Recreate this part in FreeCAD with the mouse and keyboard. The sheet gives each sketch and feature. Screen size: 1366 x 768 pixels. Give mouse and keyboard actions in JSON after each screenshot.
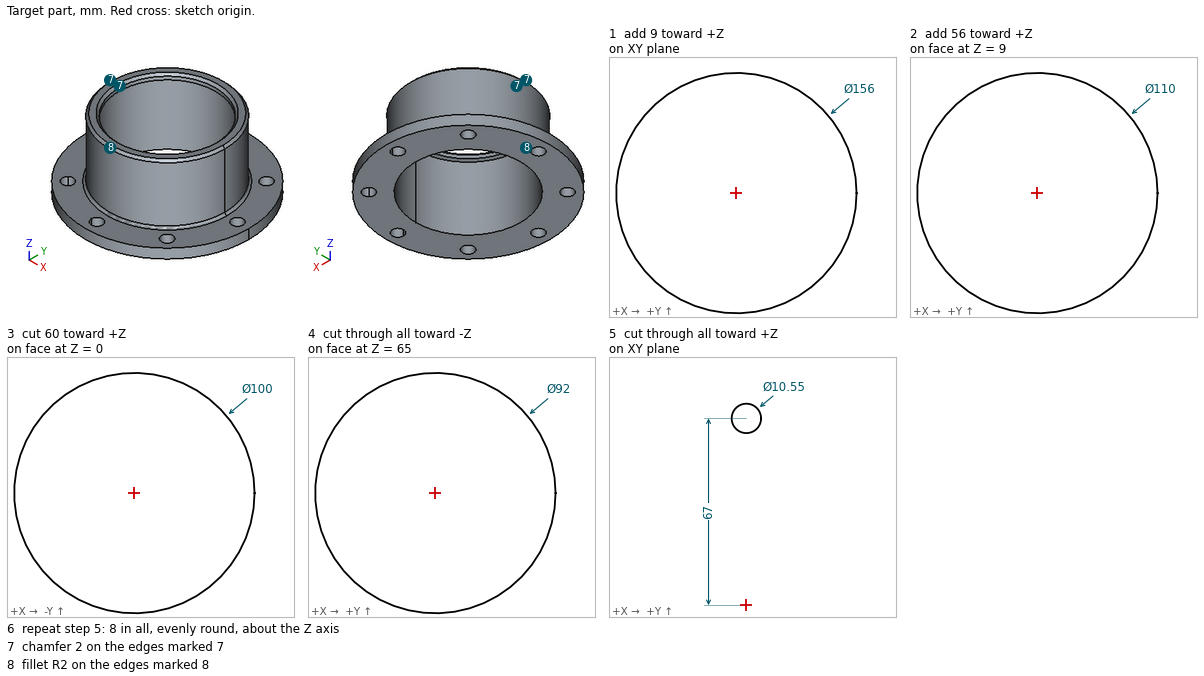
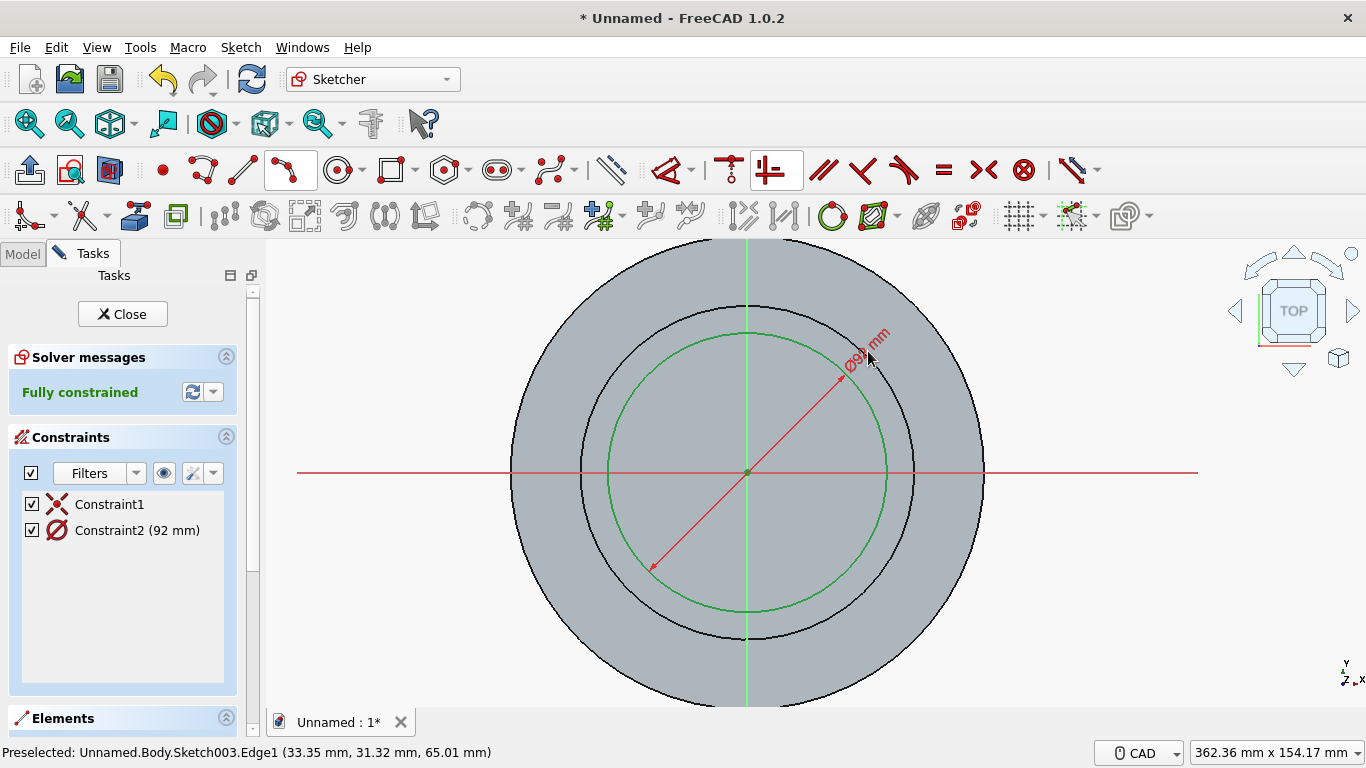
{"action": "left_click", "coordinate": [123, 314]}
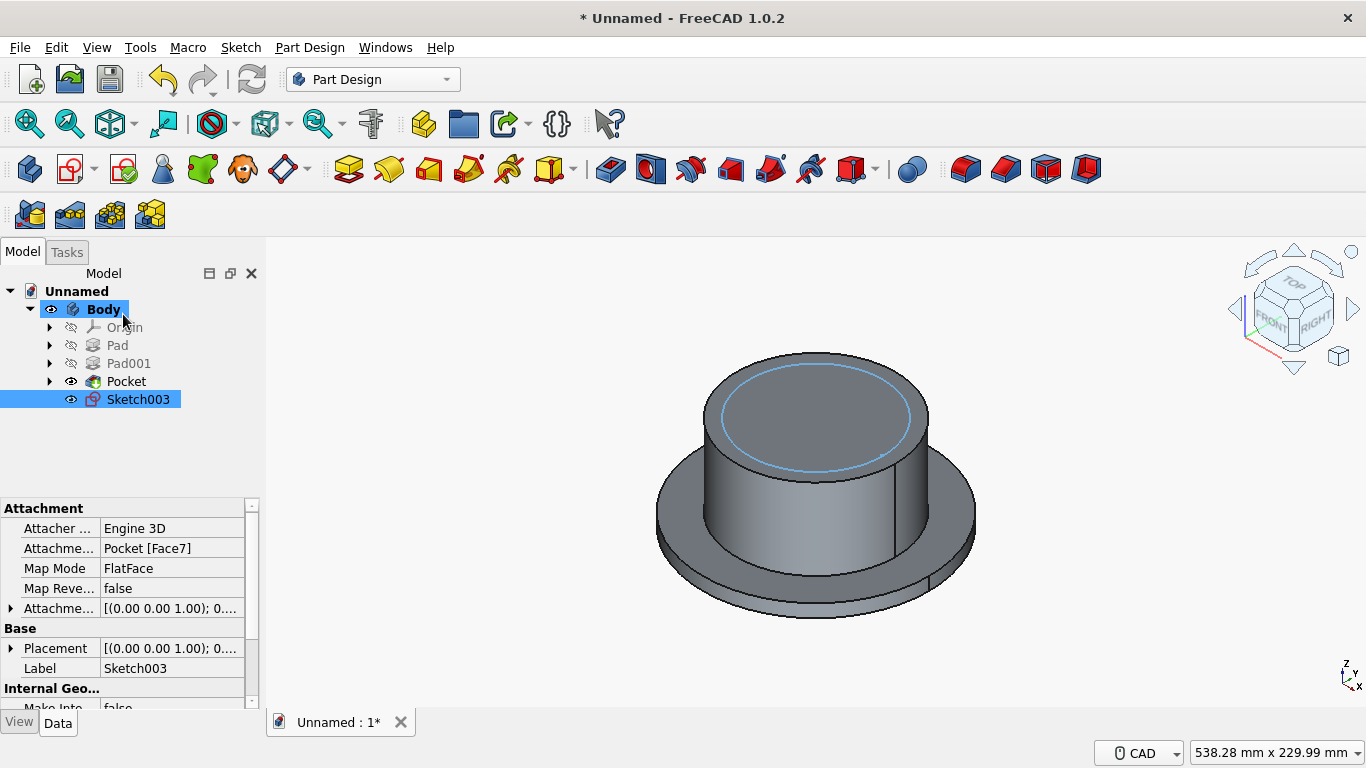
{"action": "left_click", "coordinate": [612, 170]}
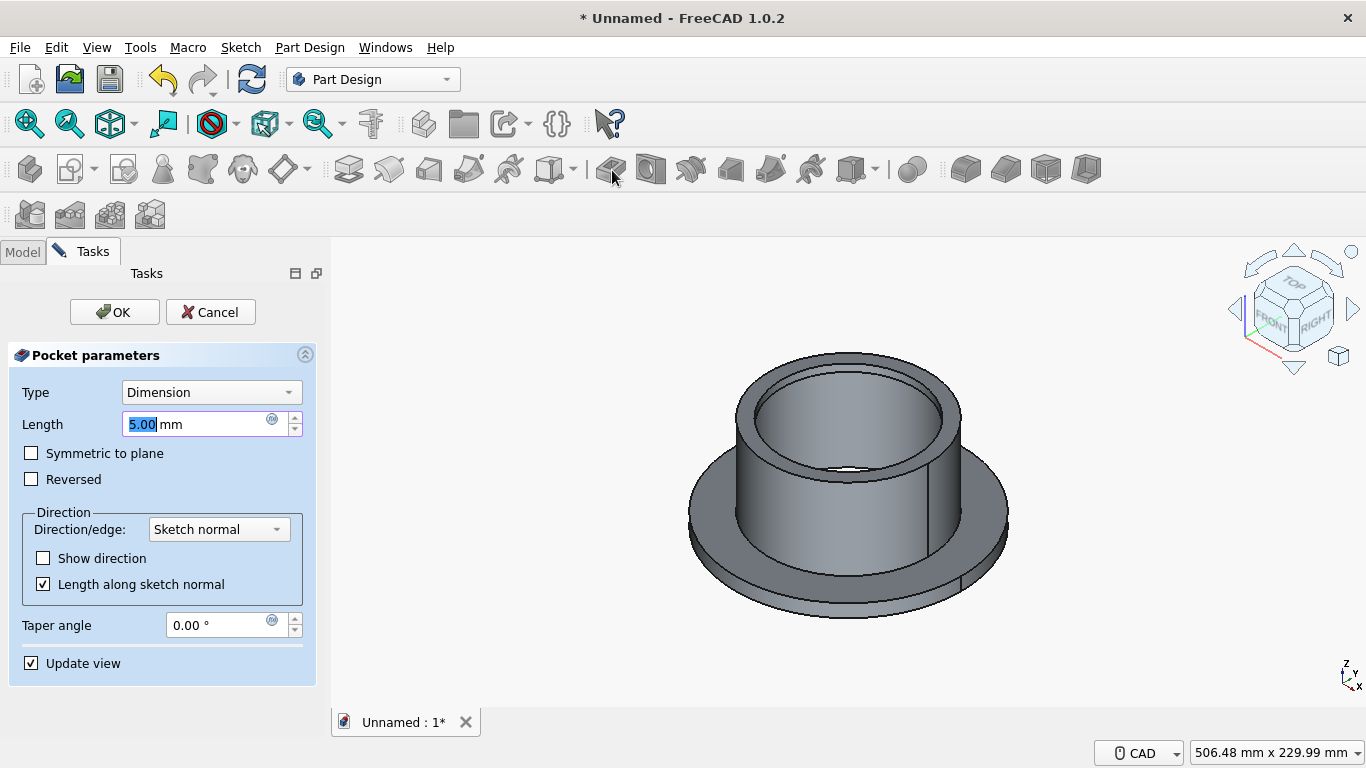
{"action": "left_click", "coordinate": [212, 392]}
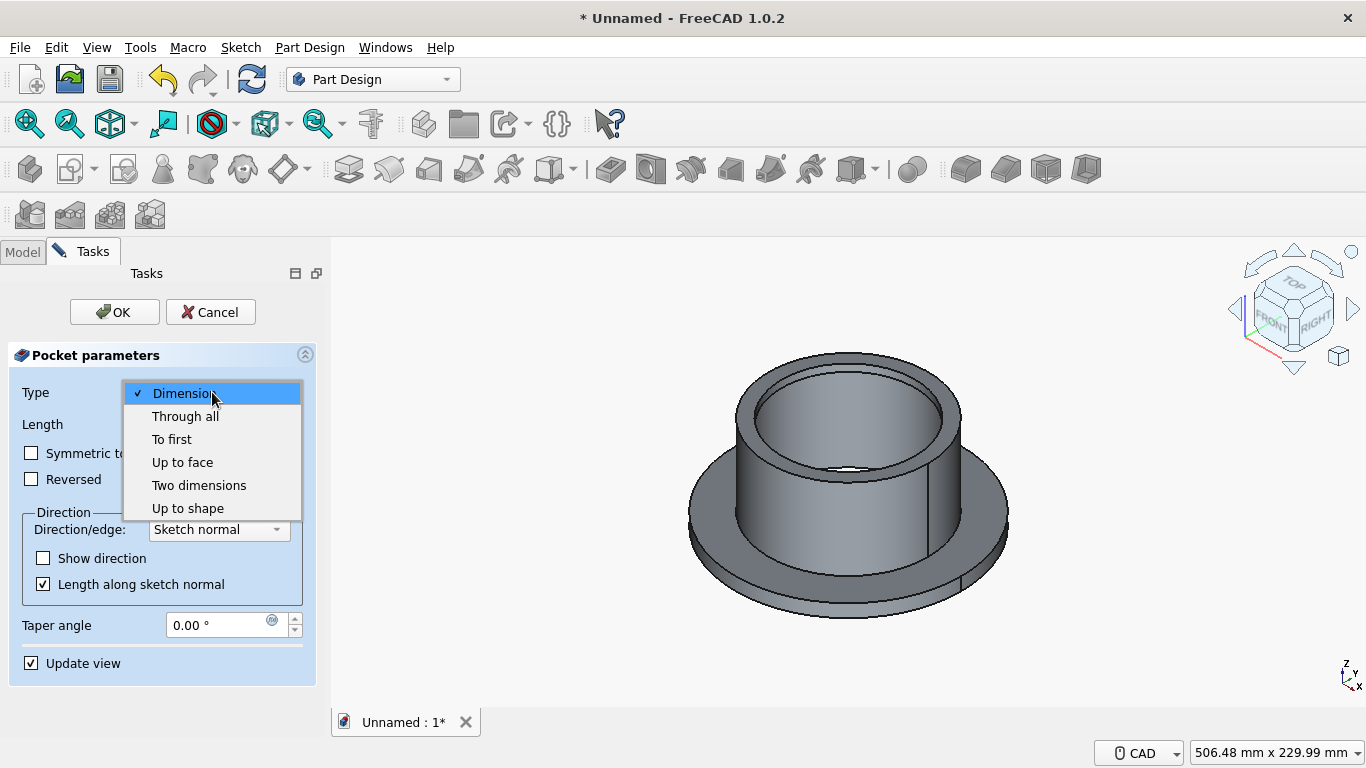
{"action": "left_click", "coordinate": [212, 416]}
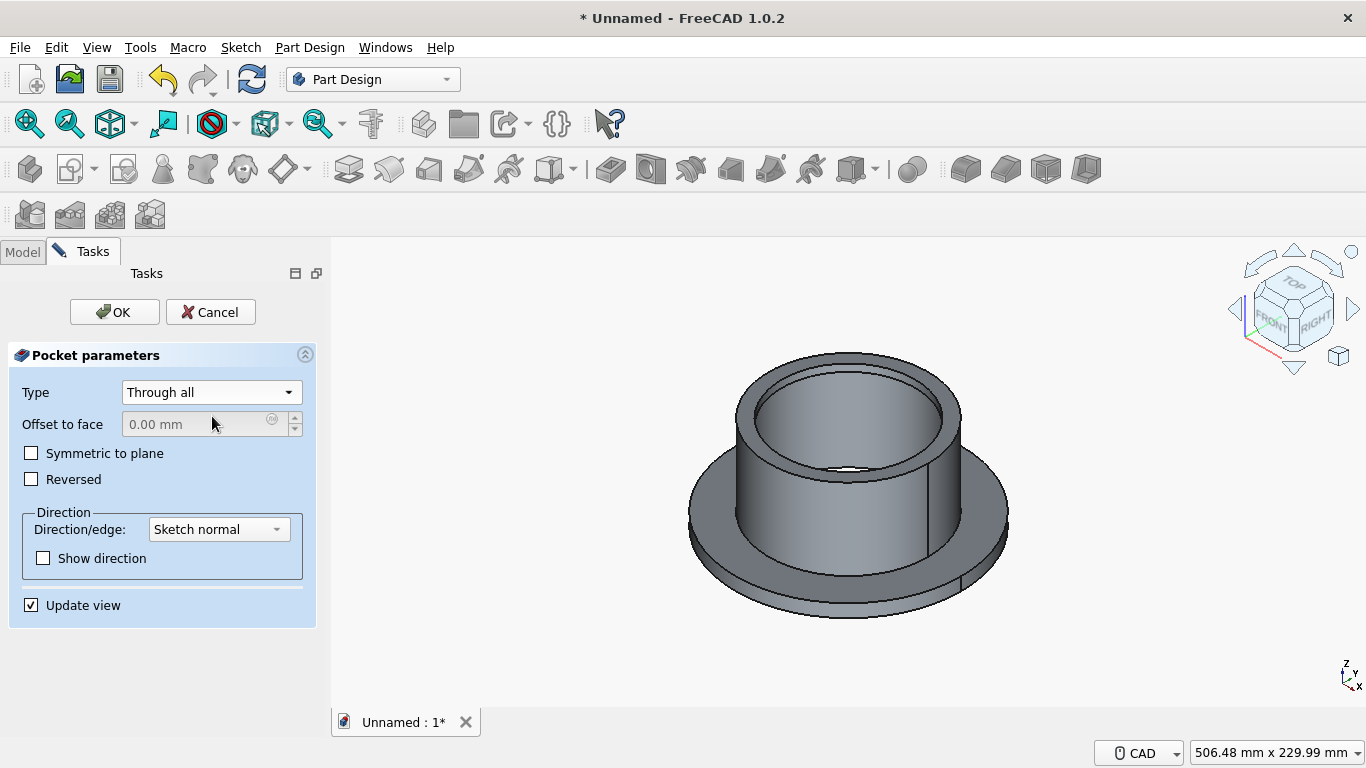
{"action": "left_click", "coordinate": [115, 312]}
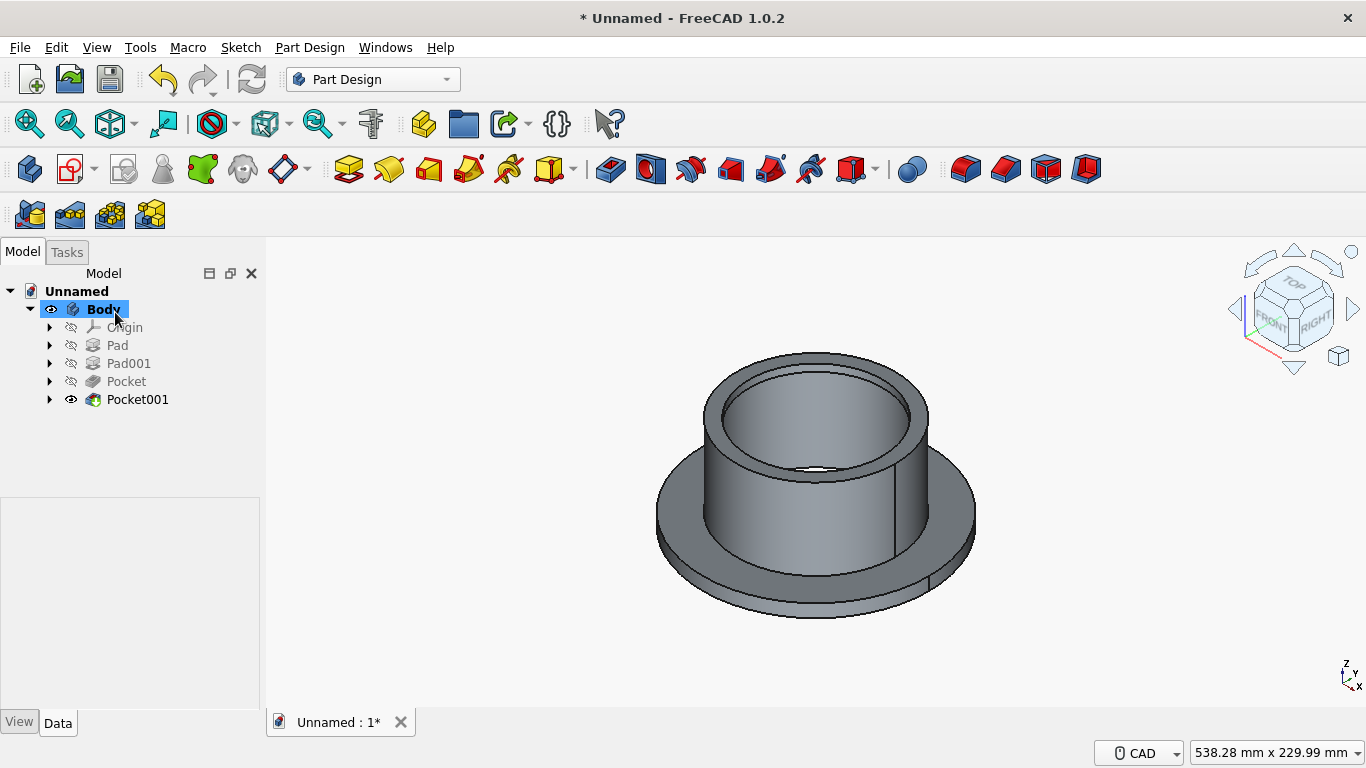
{"action": "left_click", "coordinate": [70, 170]}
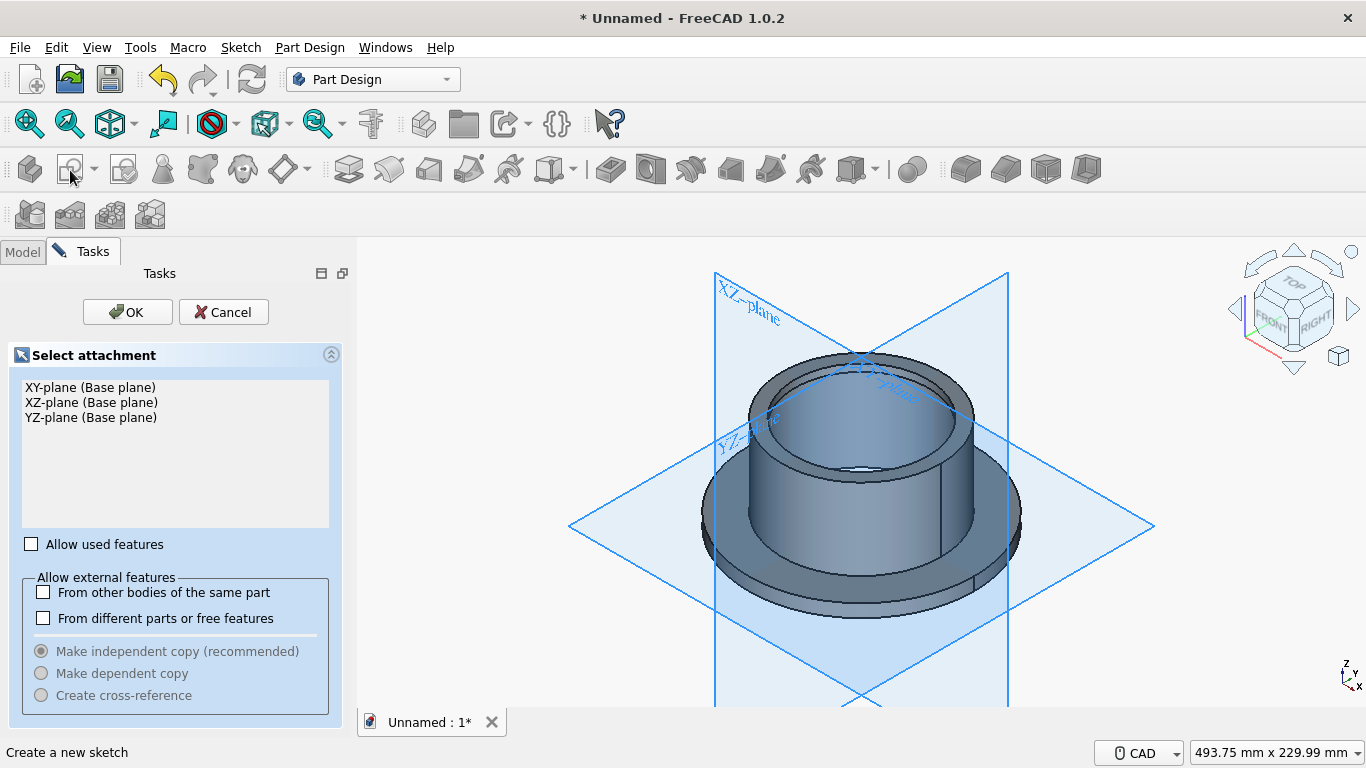
{"action": "left_click", "coordinate": [82, 388]}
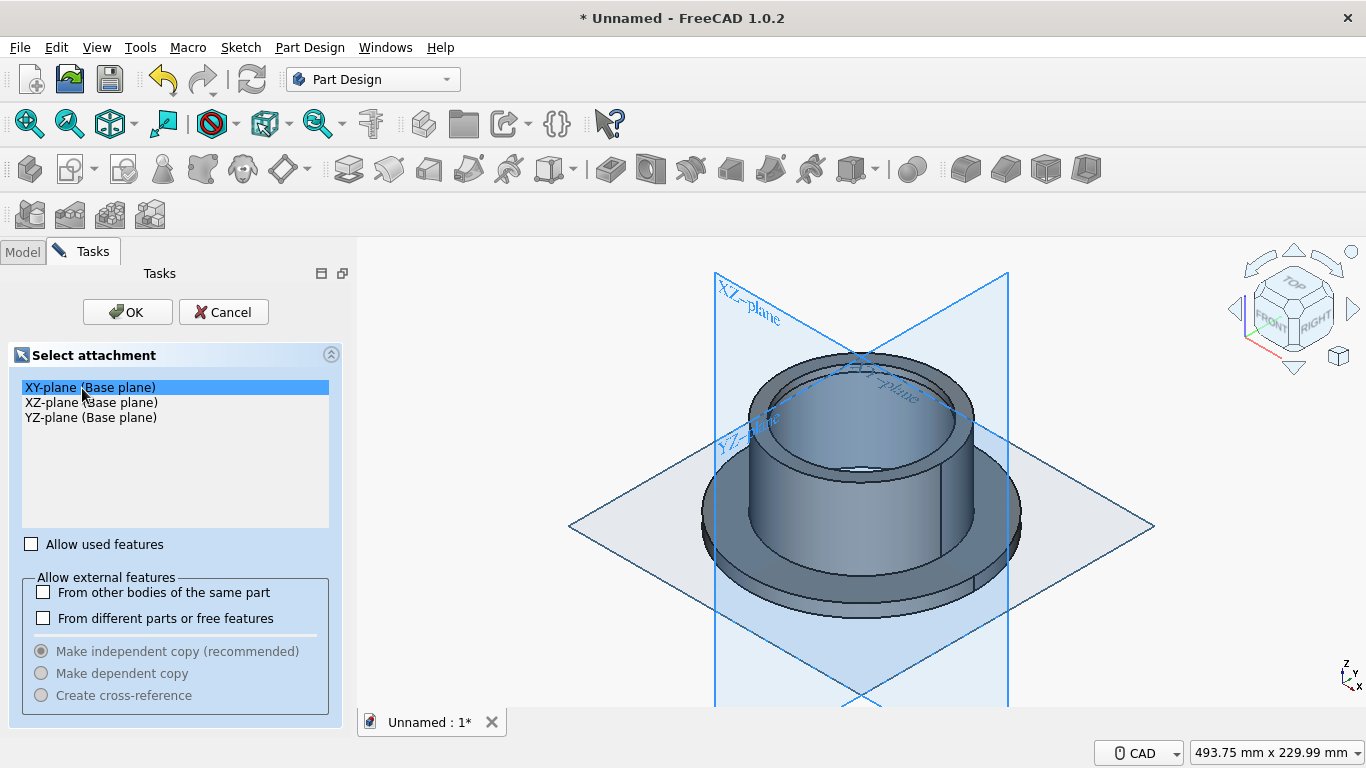
{"action": "left_click", "coordinate": [128, 312]}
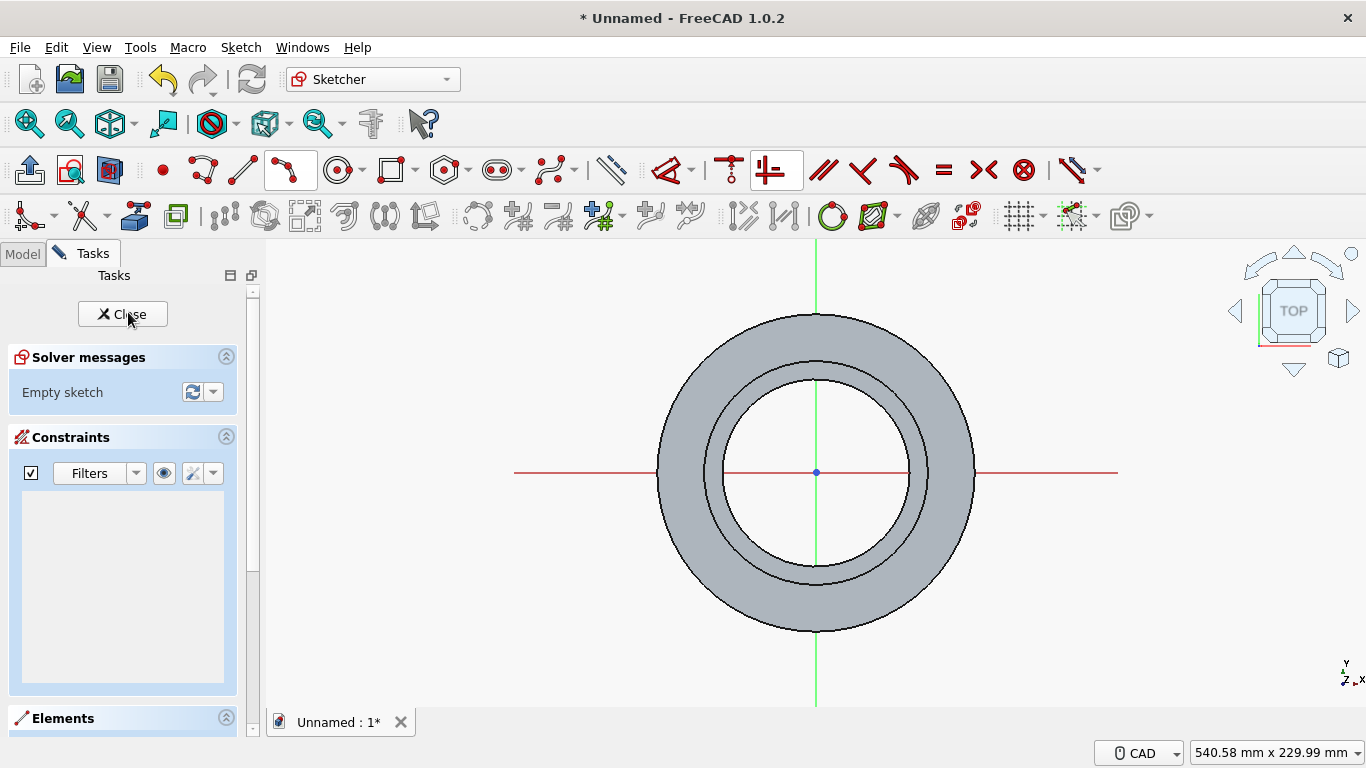
{"action": "left_click", "coordinate": [110, 170]}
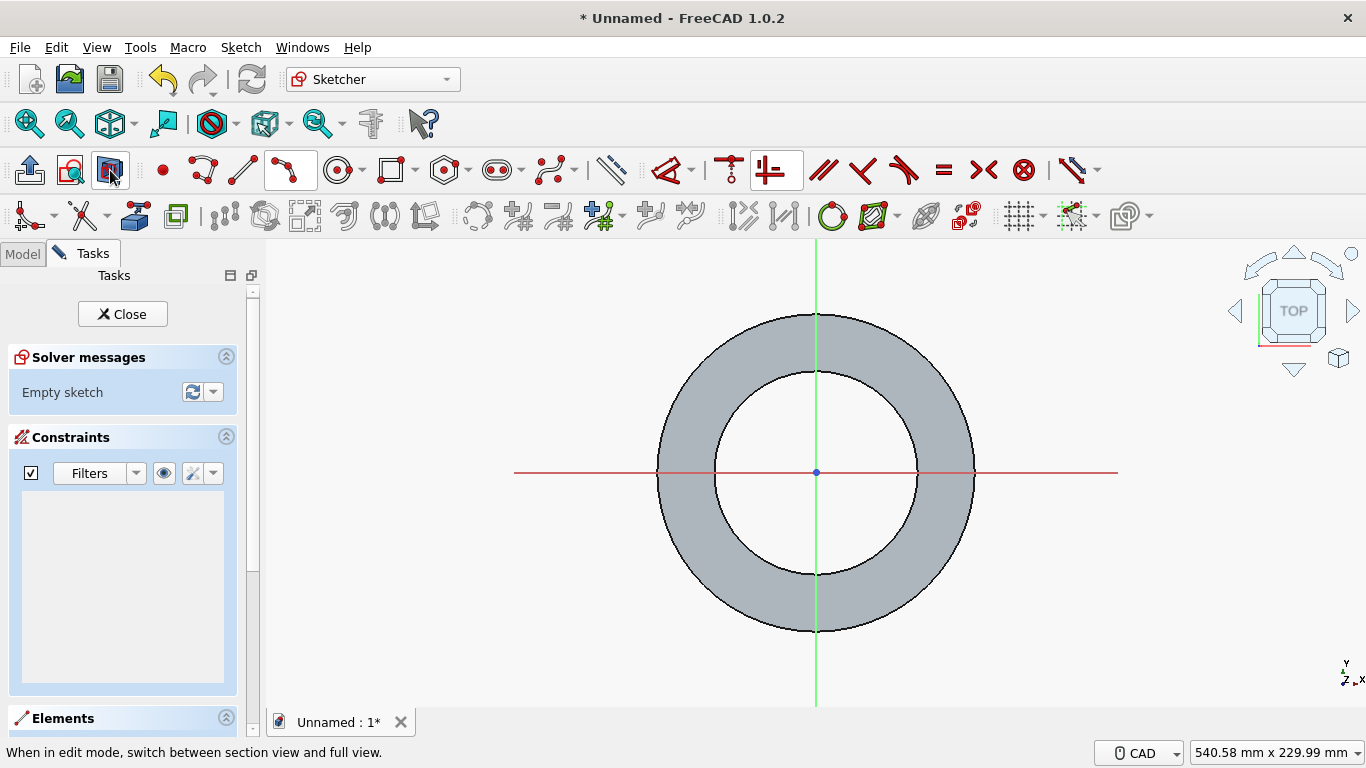
{"action": "scroll", "coordinate": [821, 326], "scroll_direction": "up", "scroll_amount": 13}